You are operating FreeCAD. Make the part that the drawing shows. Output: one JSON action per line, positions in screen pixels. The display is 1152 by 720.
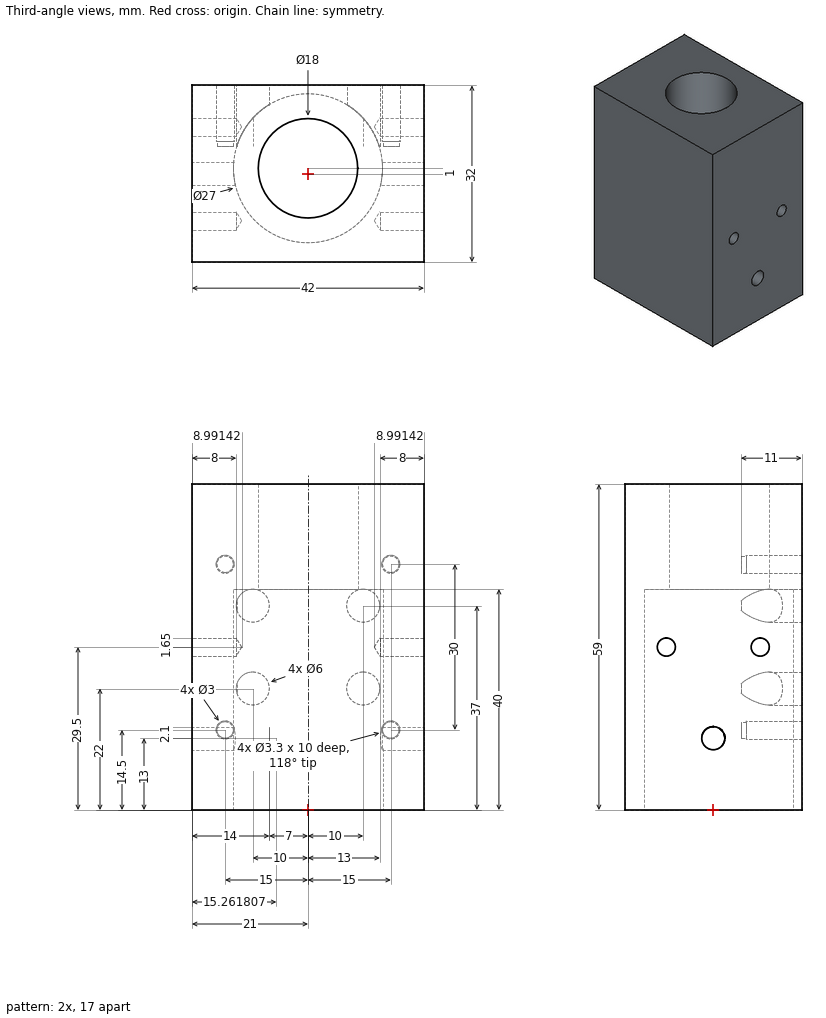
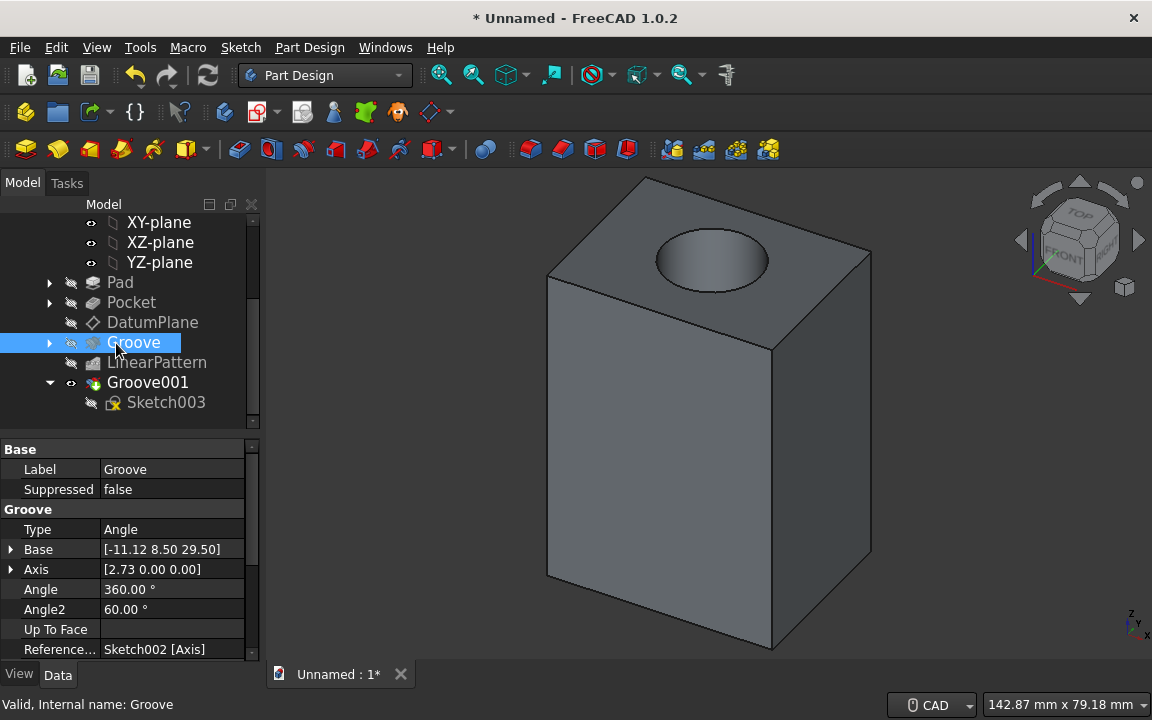
{"action": "left_click", "coordinate": [116, 383], "text": "ctrl"}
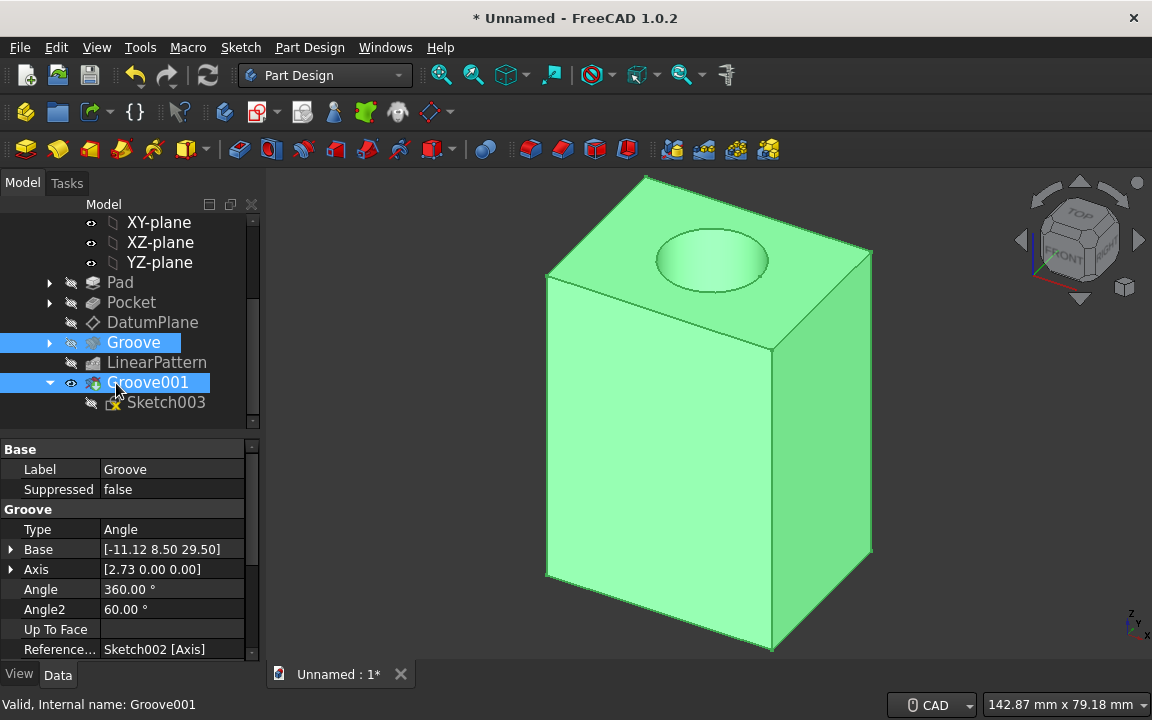
{"action": "left_click", "coordinate": [672, 150]}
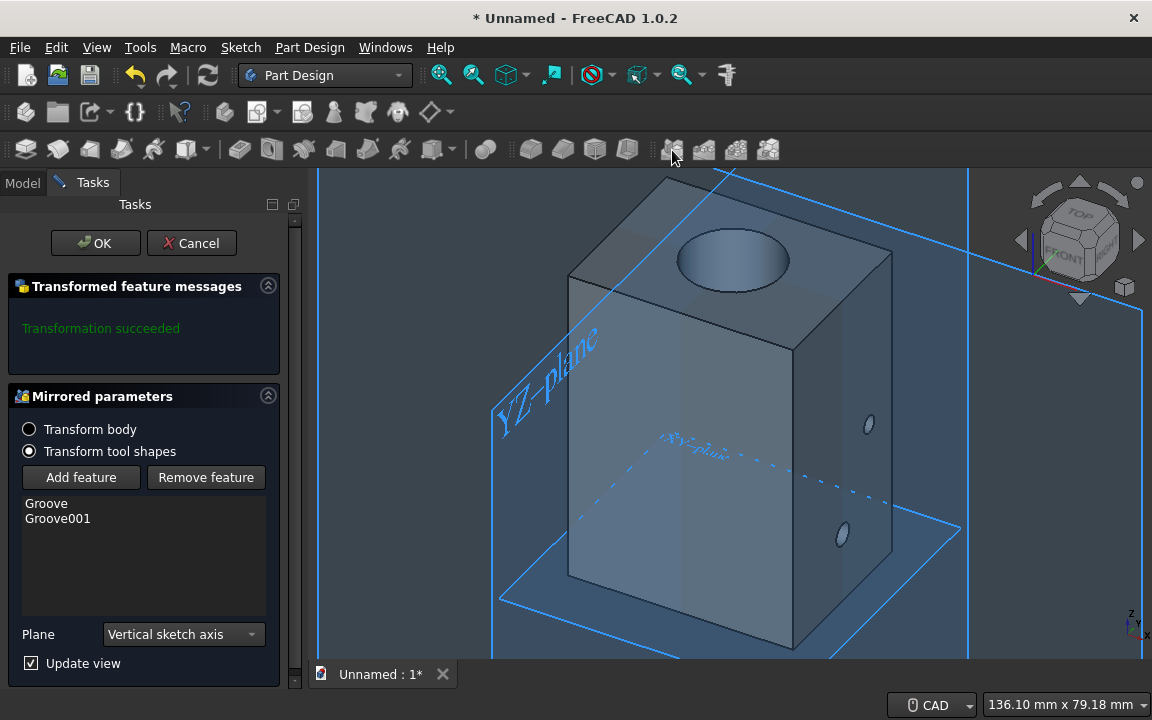
{"action": "left_click", "coordinate": [184, 634]}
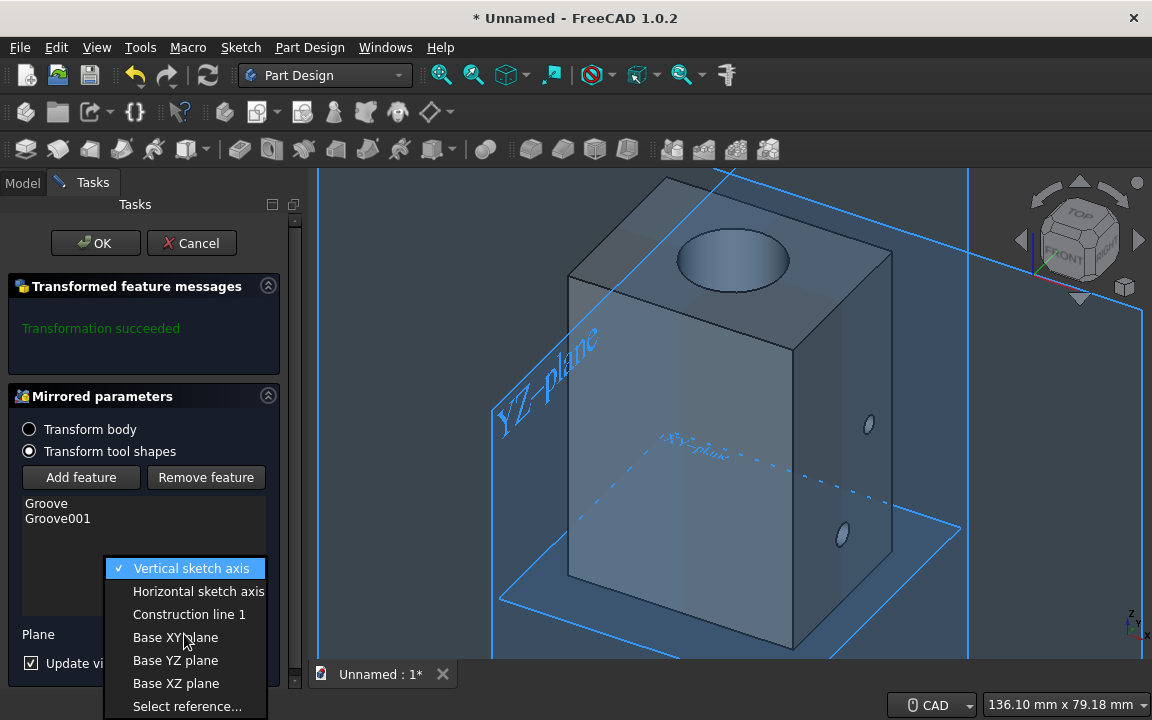
{"action": "left_click", "coordinate": [184, 660]}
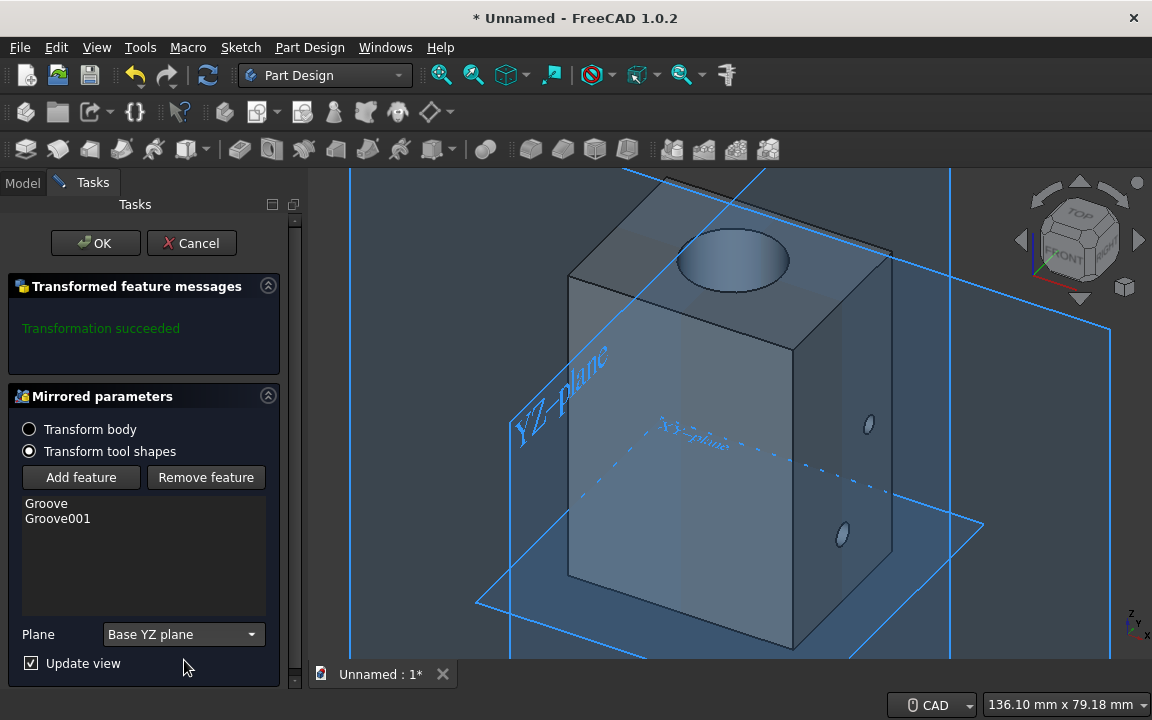
{"action": "left_click", "coordinate": [96, 243]}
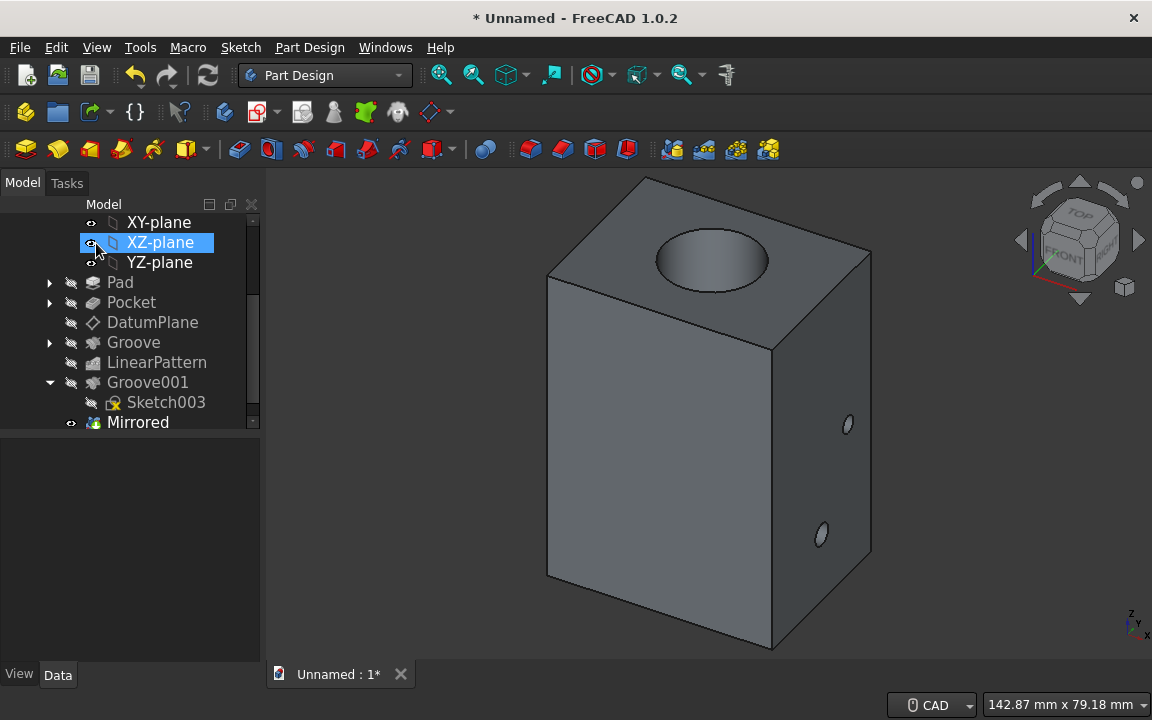
{"action": "scroll", "coordinate": [160, 318], "scroll_direction": "down", "scroll_amount": 3}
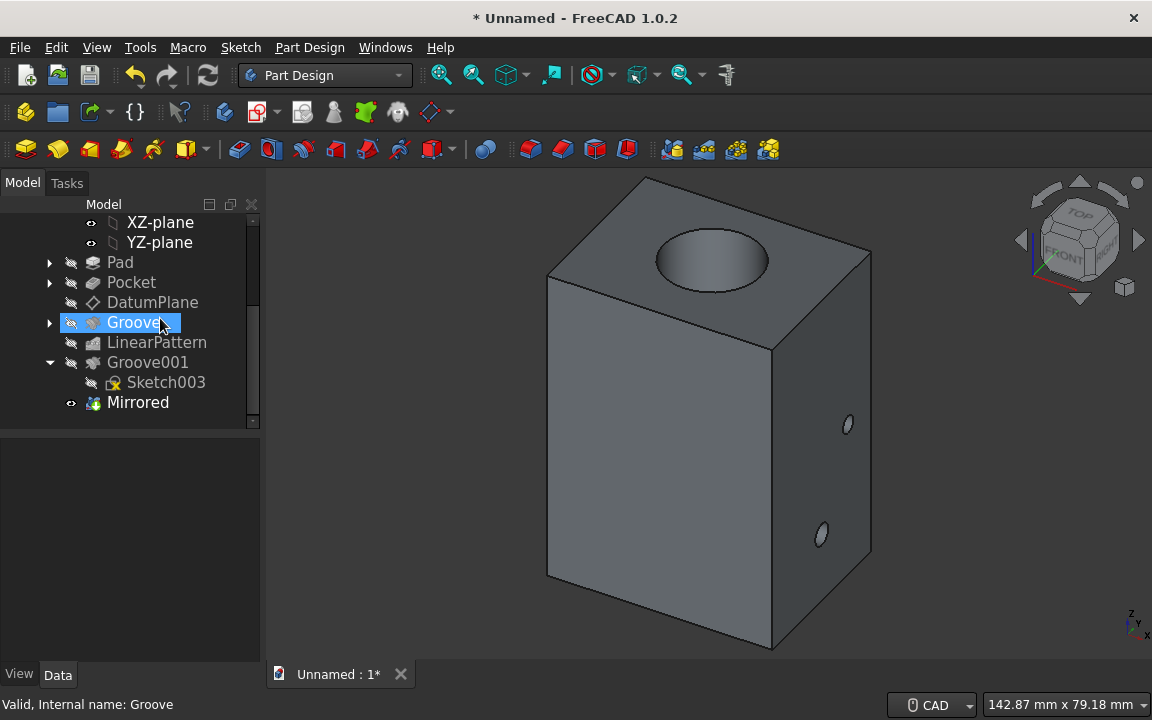
{"action": "scroll", "coordinate": [160, 318], "scroll_direction": "up", "scroll_amount": 15}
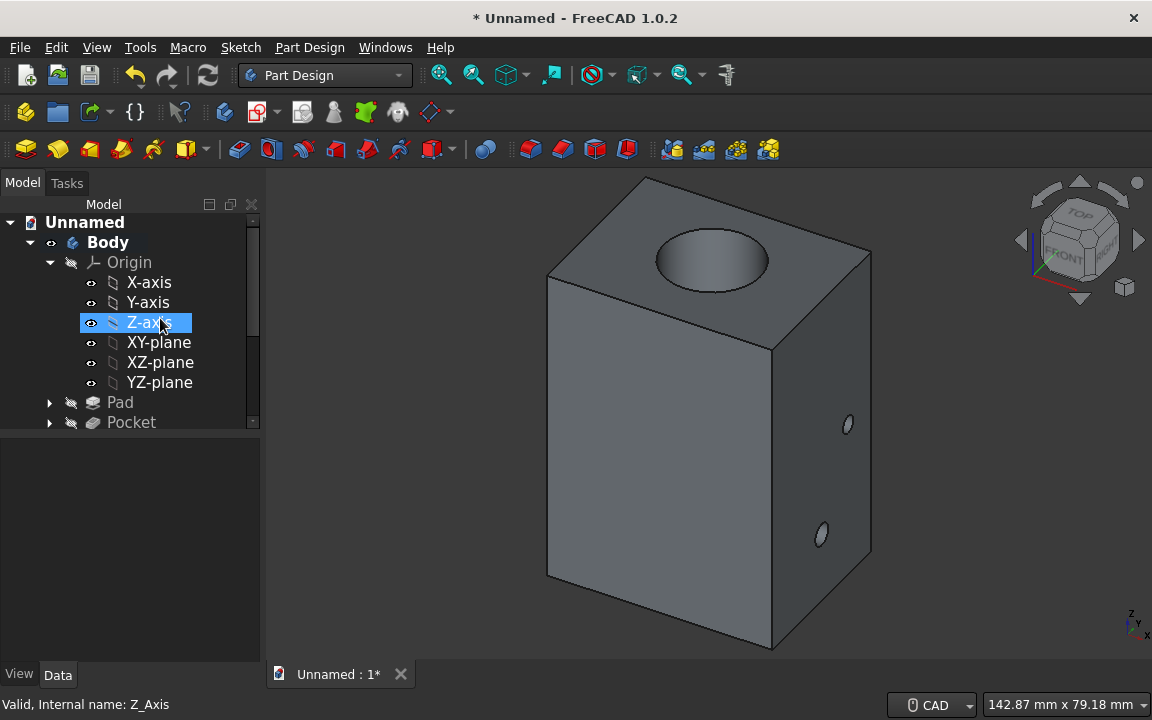
{"action": "left_click", "coordinate": [136, 363]}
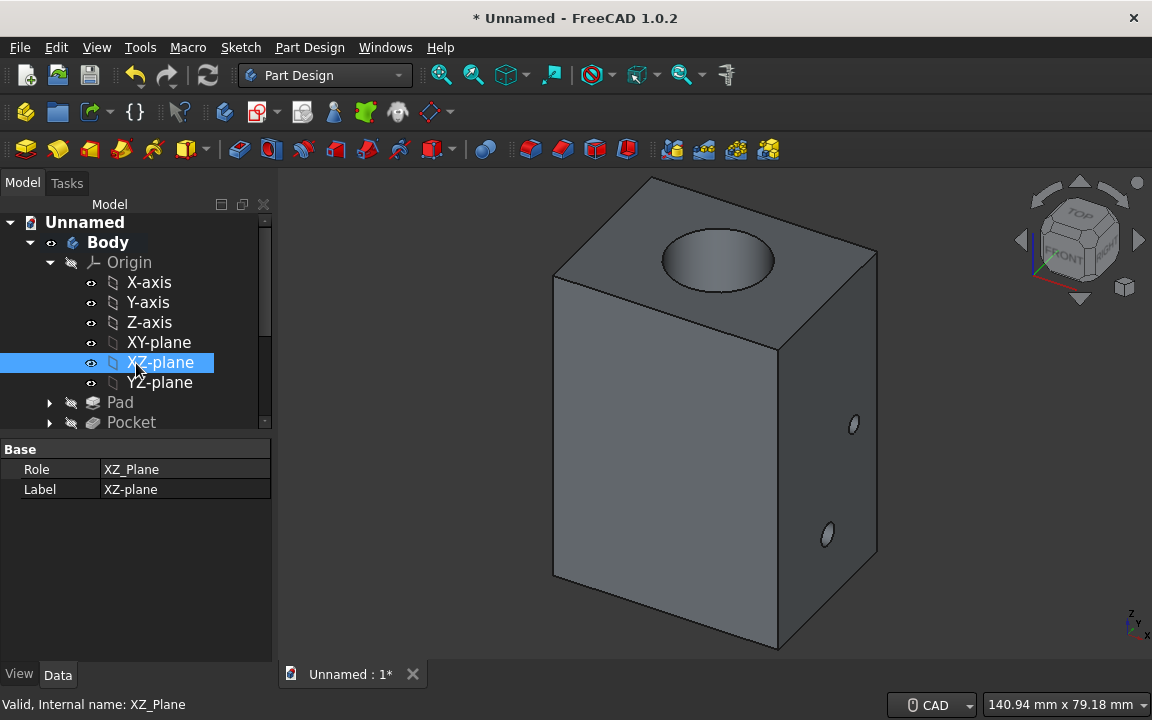
{"action": "left_click", "coordinate": [430, 112]}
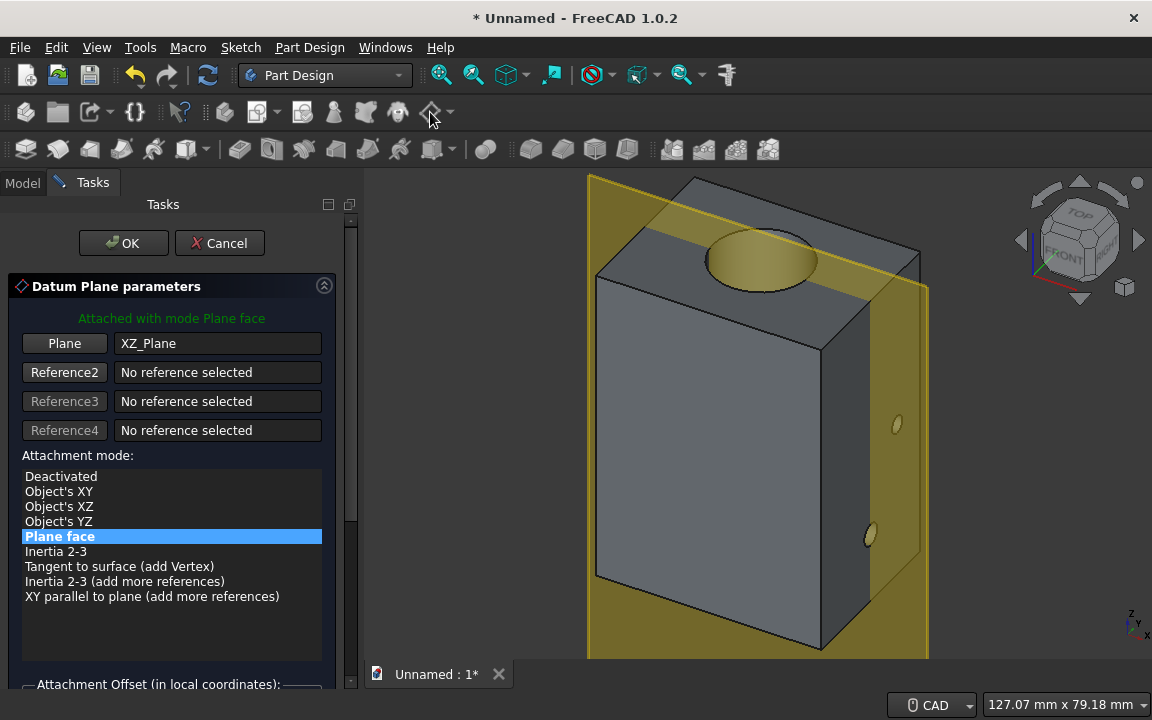
{"action": "scroll", "coordinate": [351, 451], "scroll_direction": "down", "scroll_amount": 3}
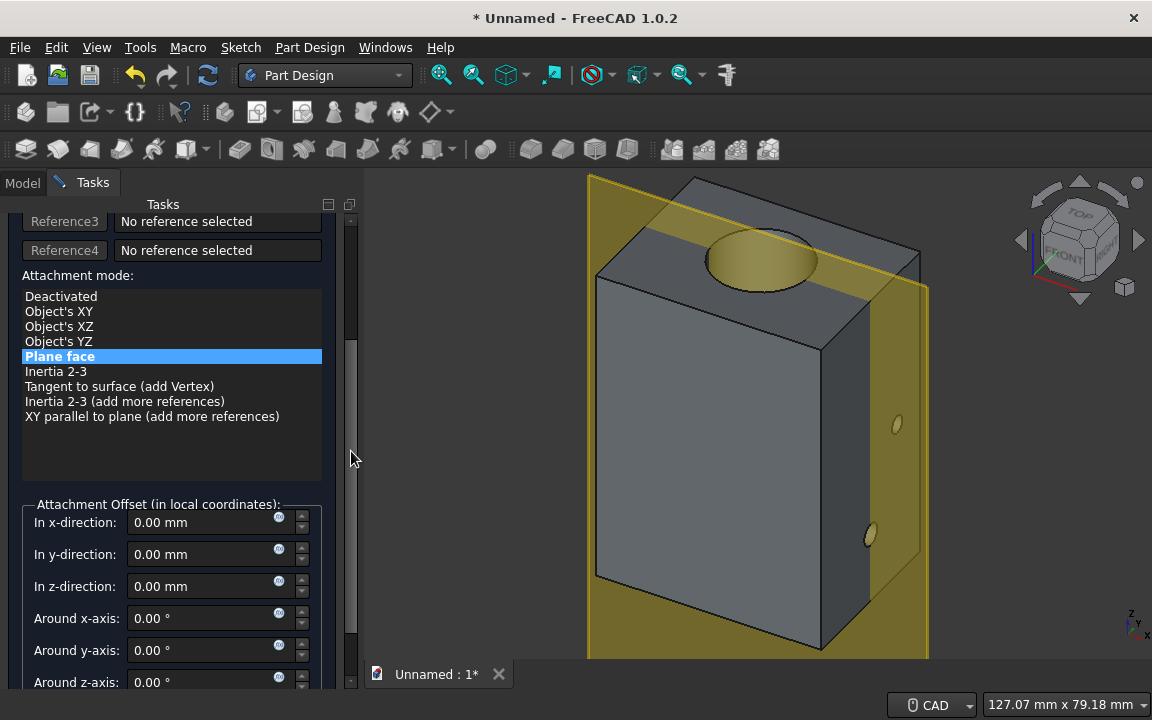
{"action": "triple_click", "coordinate": [210, 586]}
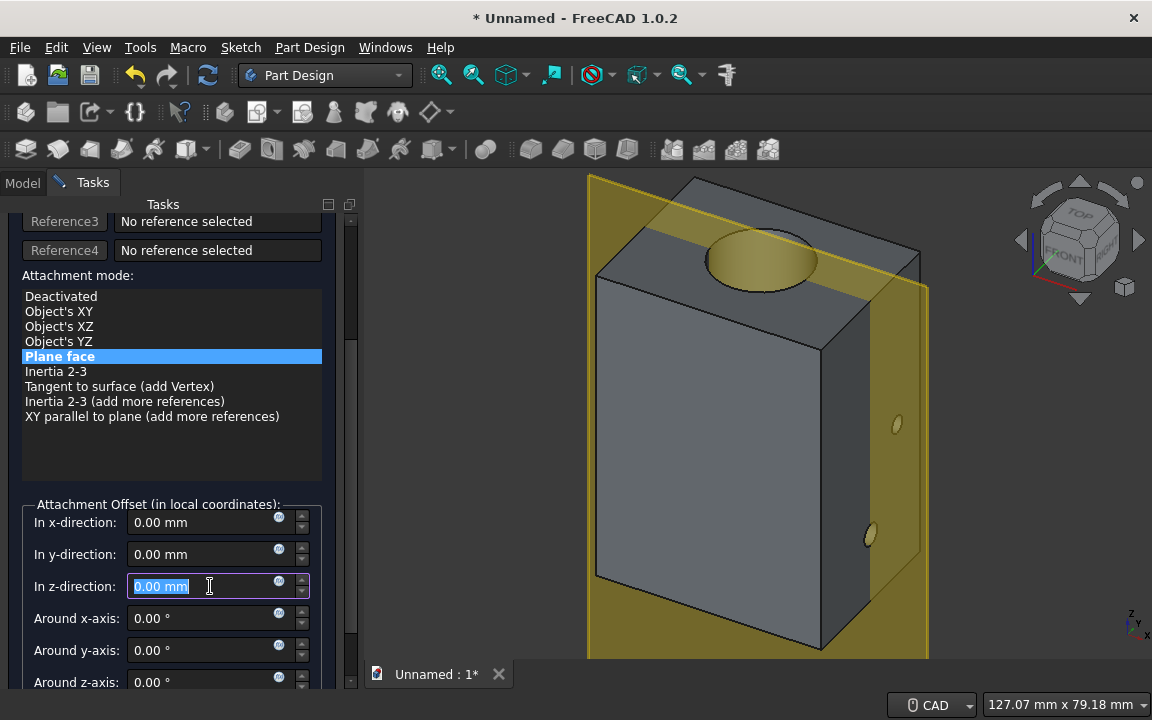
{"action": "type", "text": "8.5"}
{"action": "key", "text": "Tab"}